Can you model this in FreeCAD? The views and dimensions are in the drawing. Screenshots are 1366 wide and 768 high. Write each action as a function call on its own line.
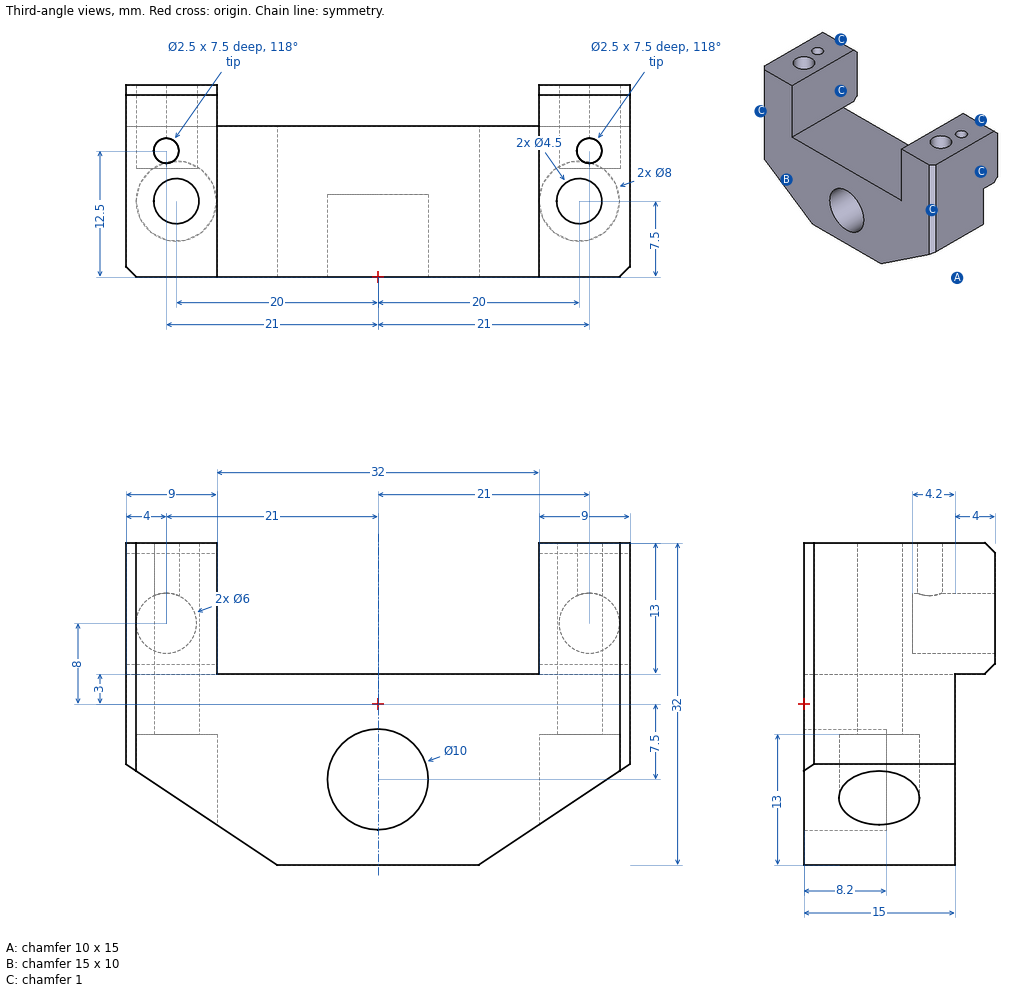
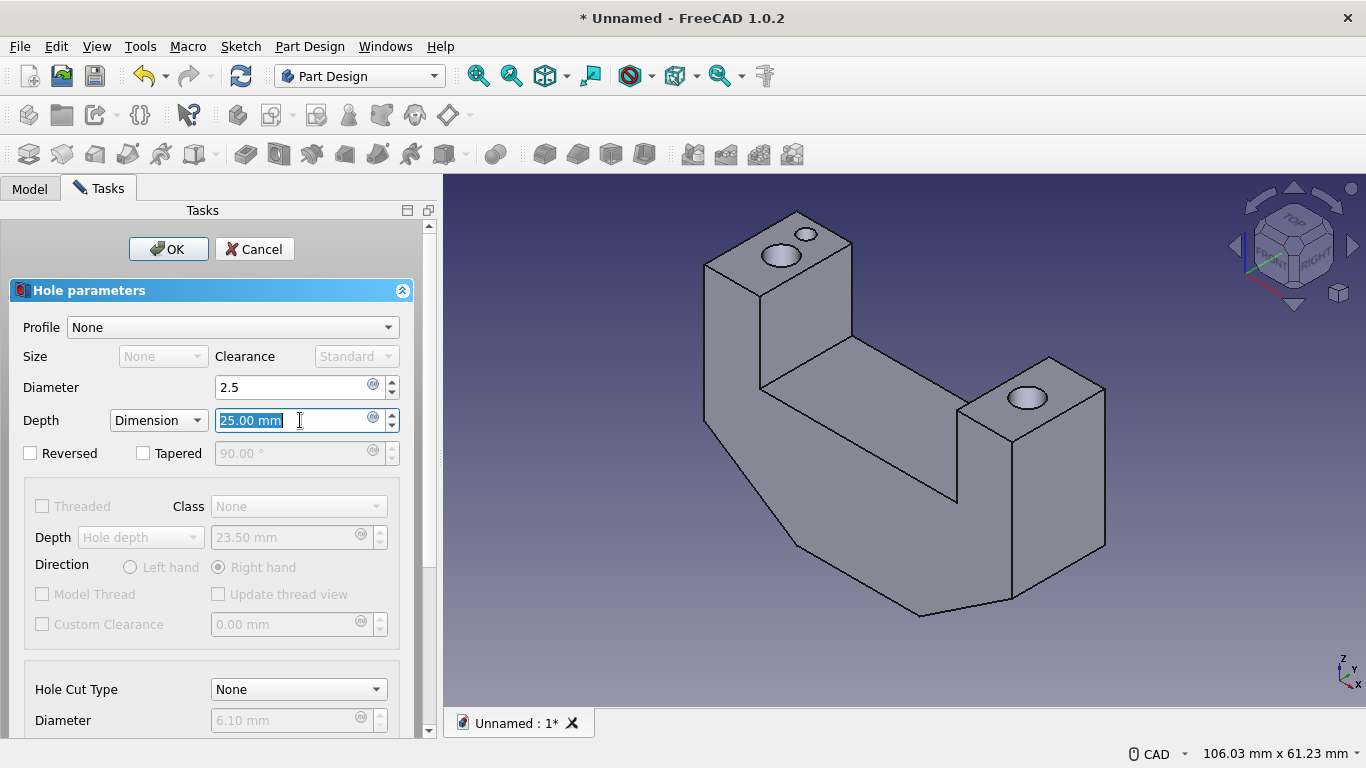
text(7.5)
key(Tab)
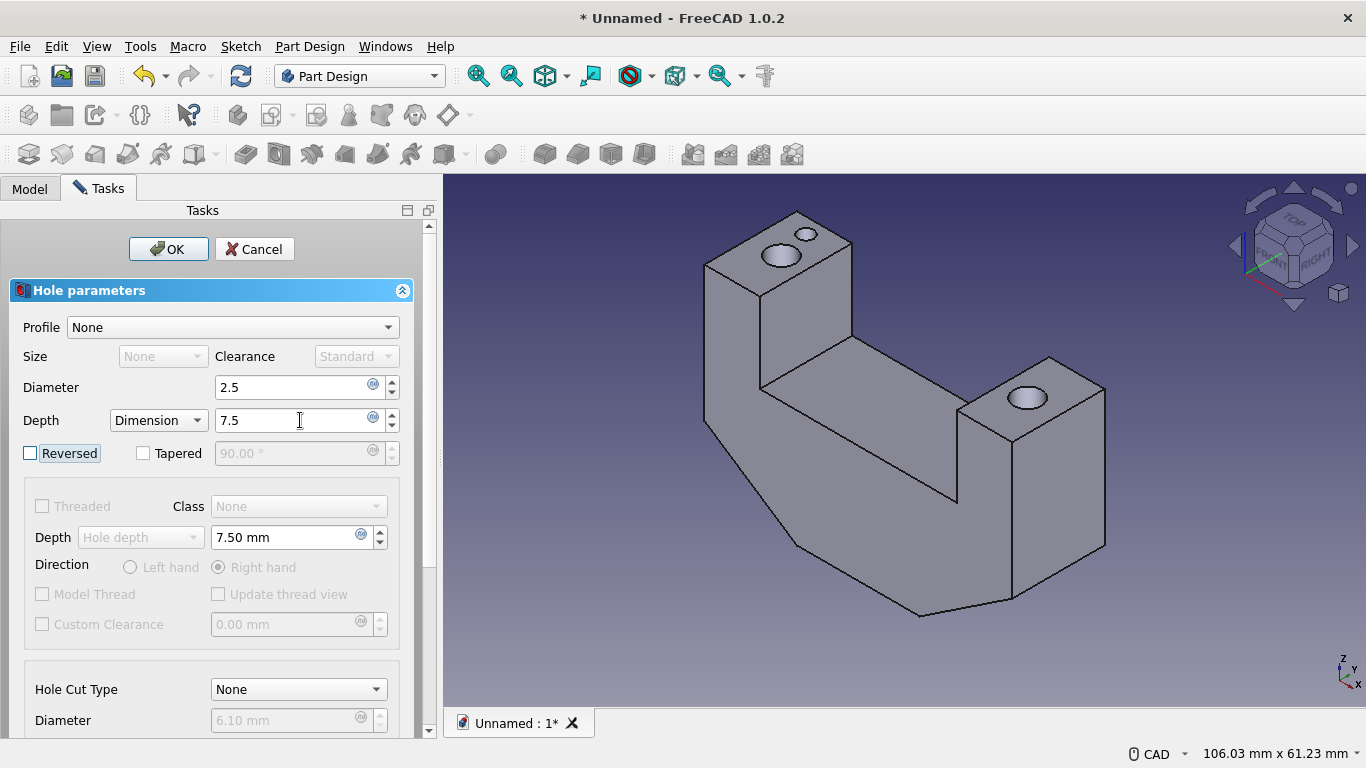
click(169, 249)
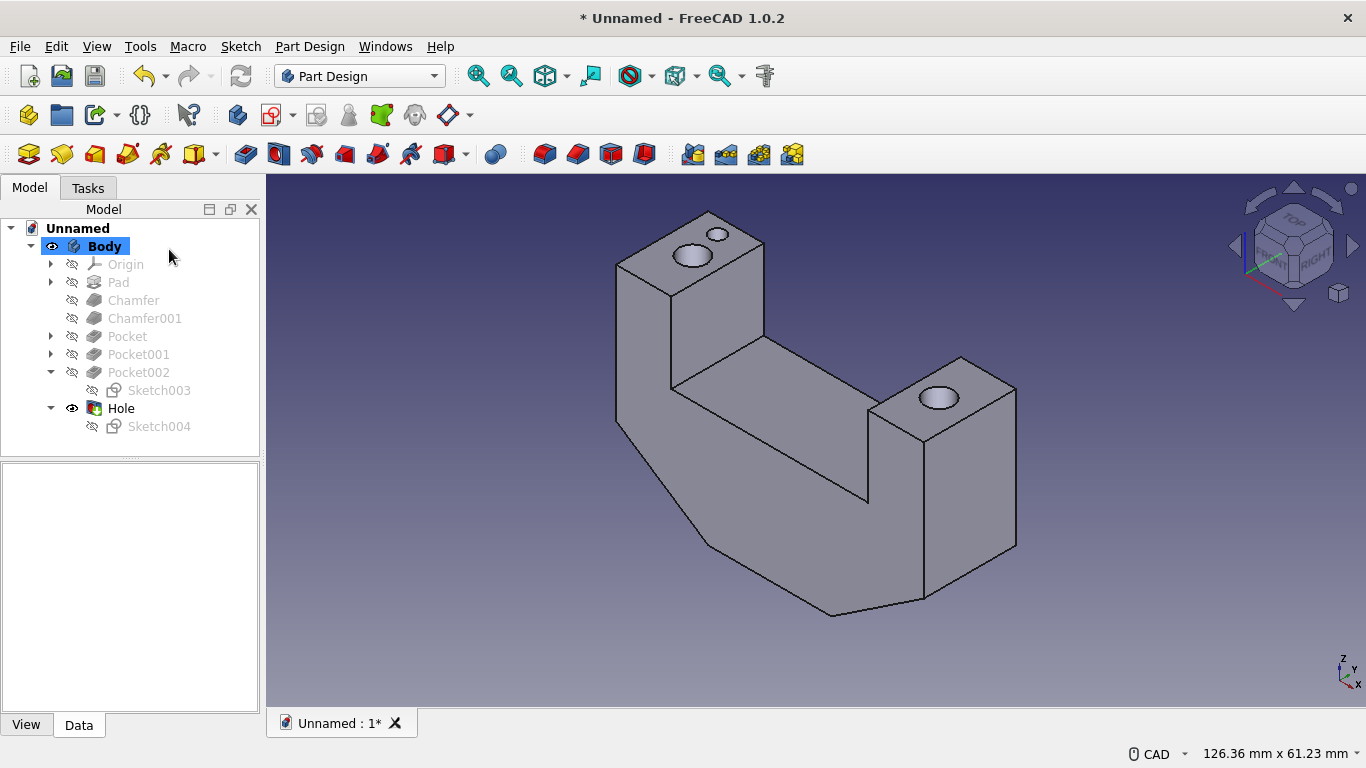
click(976, 388)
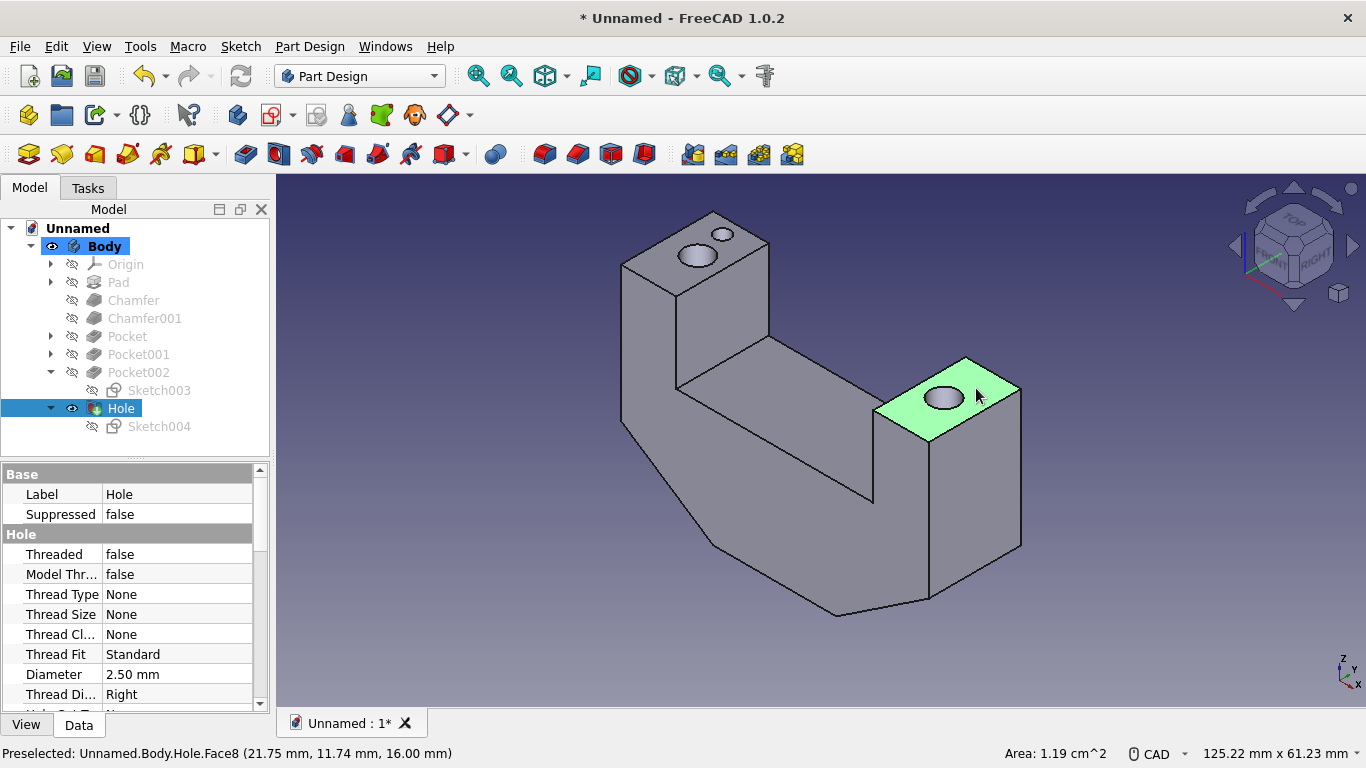
click(270, 116)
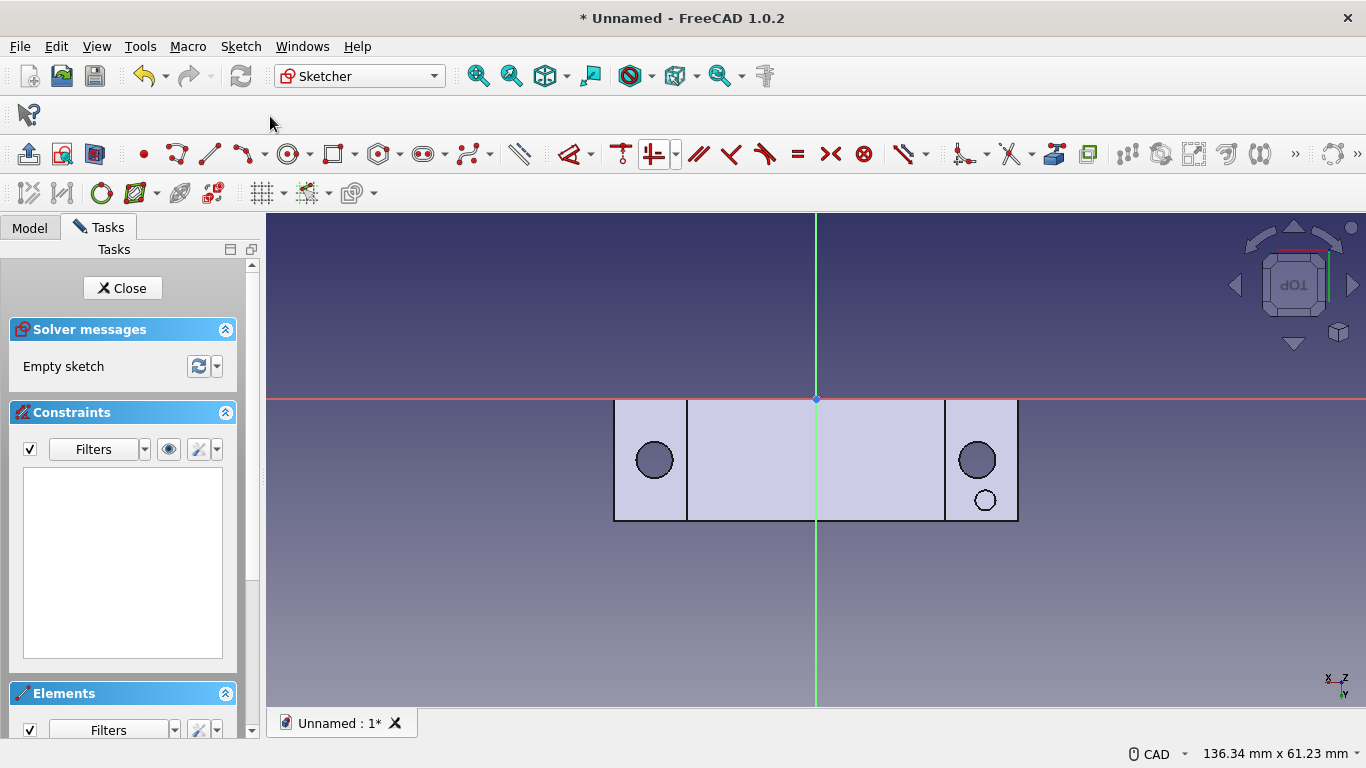
scroll(640, 503, up, 14)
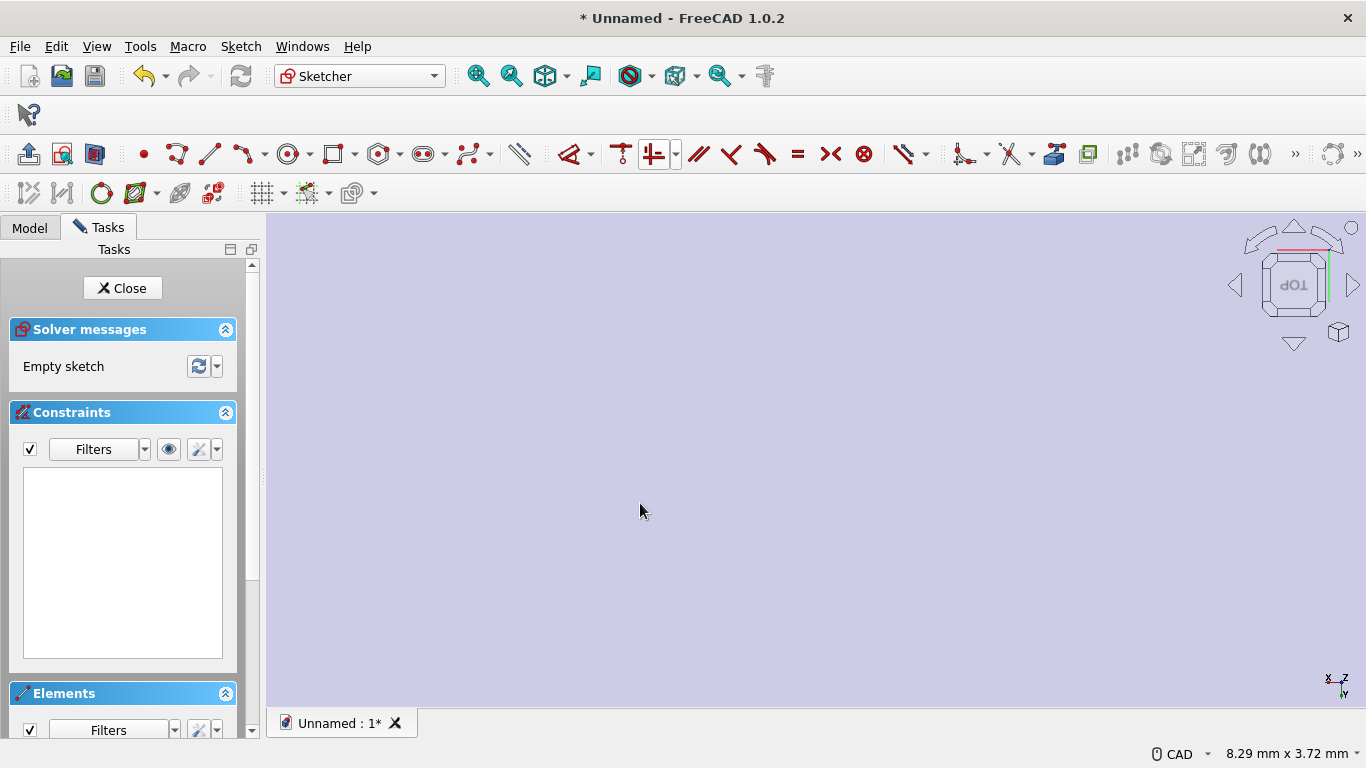
click(288, 154)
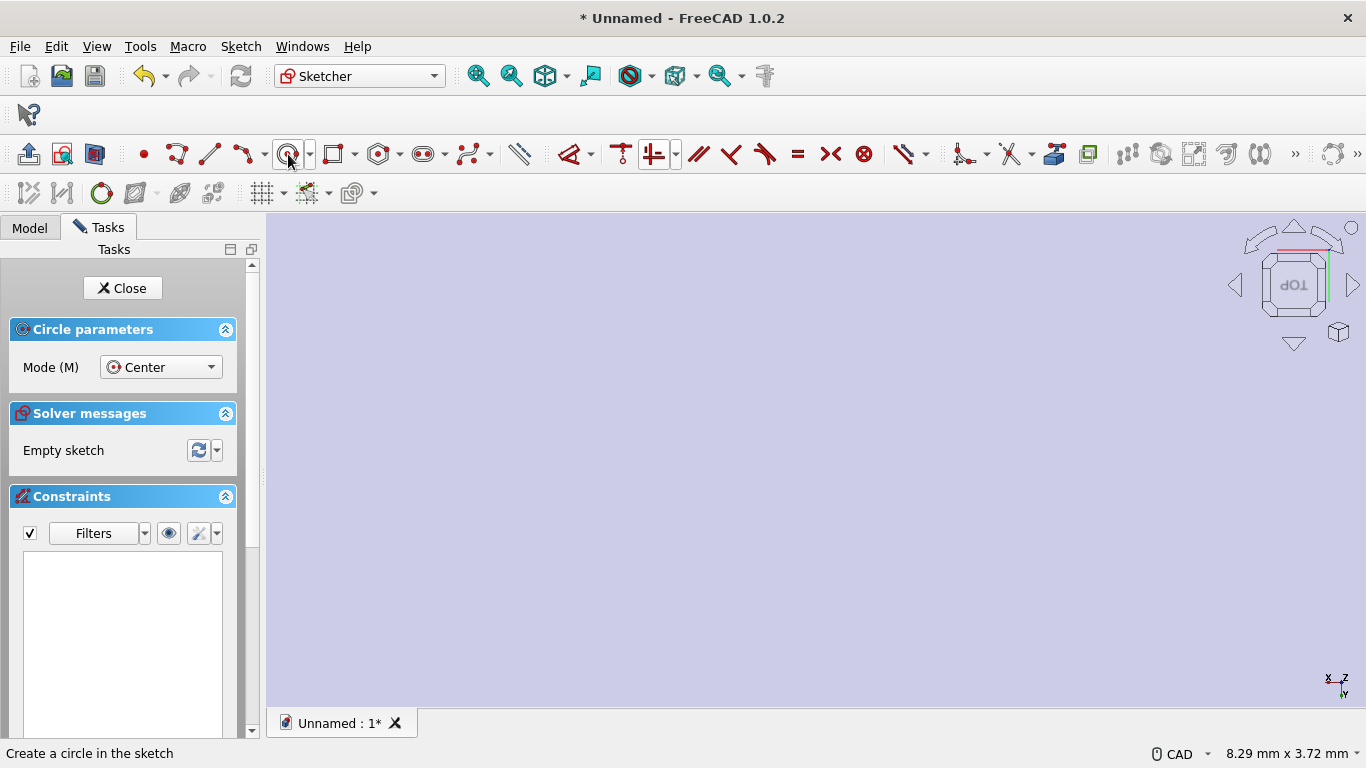
click(743, 450)
move(860, 333)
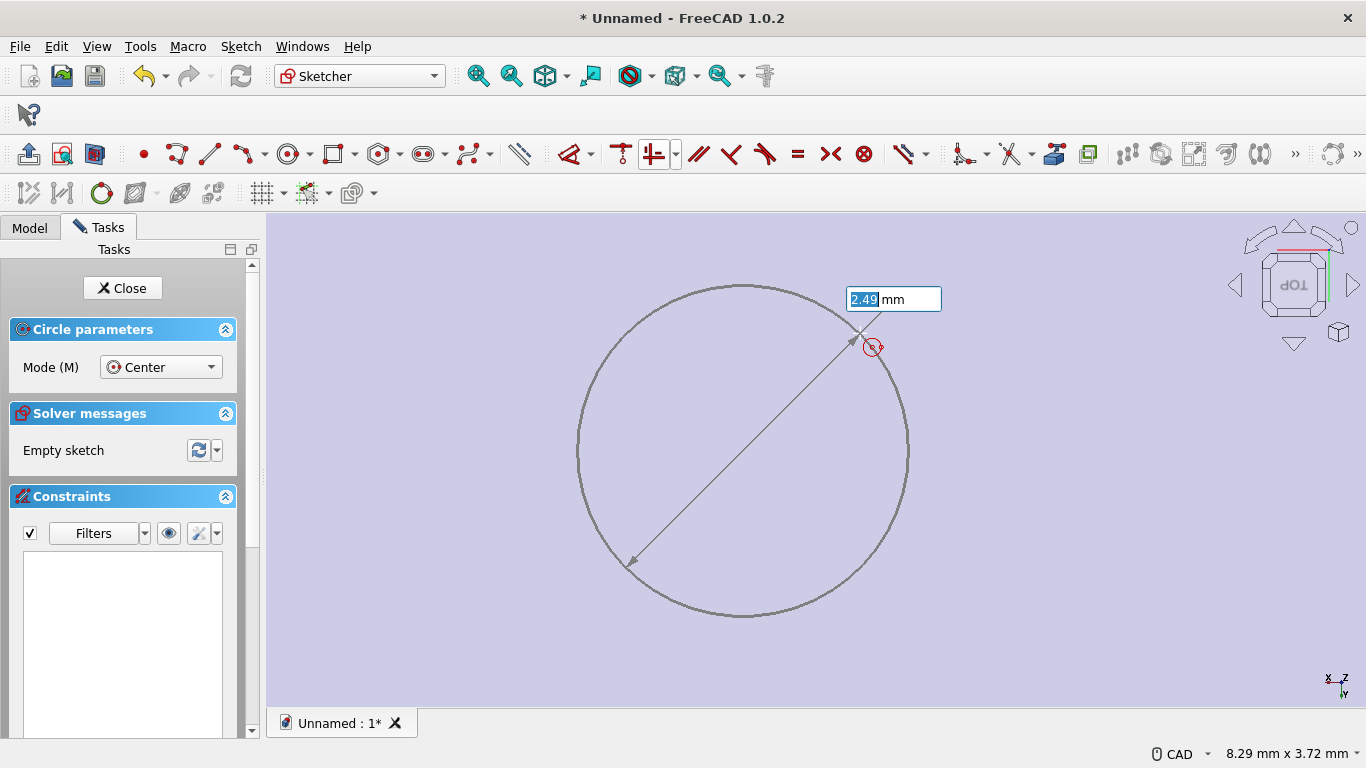
text(2.5)
key(Return)
key(Escape)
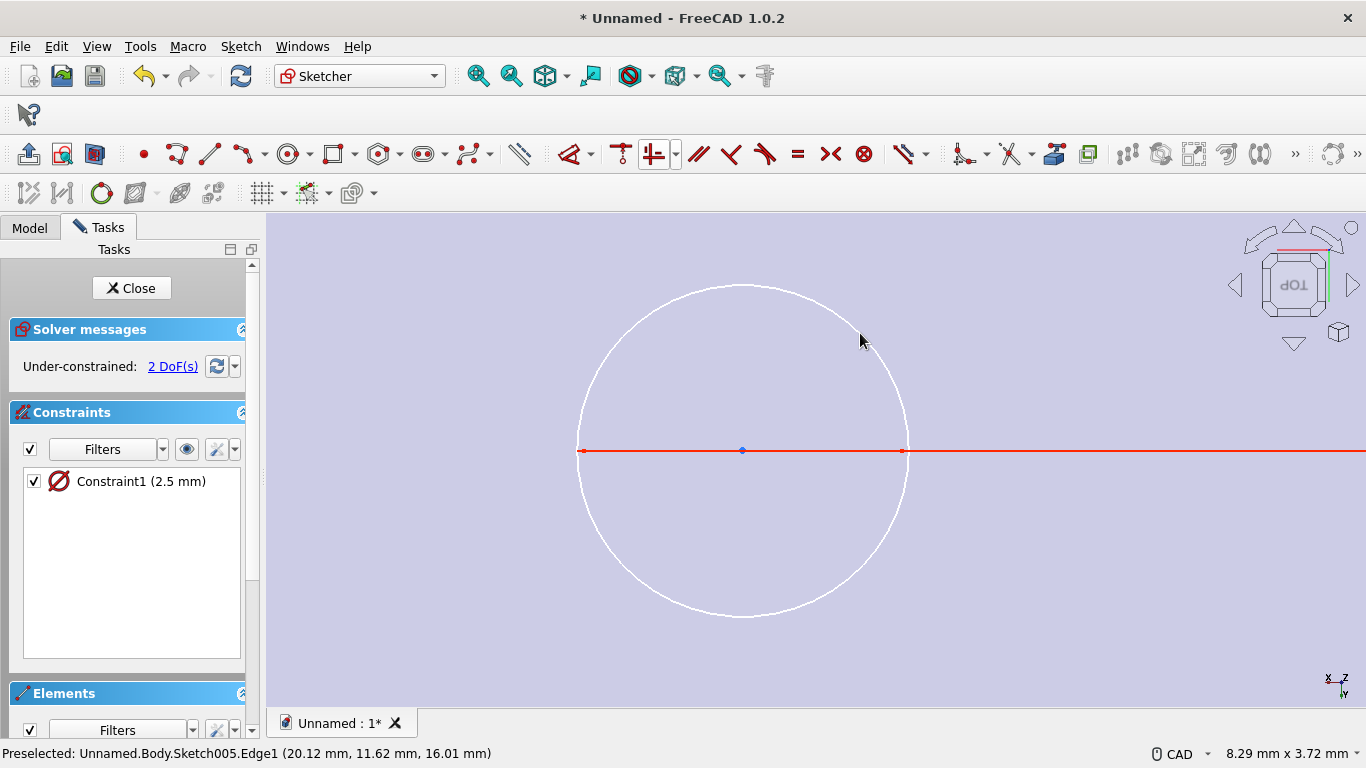
click(568, 154)